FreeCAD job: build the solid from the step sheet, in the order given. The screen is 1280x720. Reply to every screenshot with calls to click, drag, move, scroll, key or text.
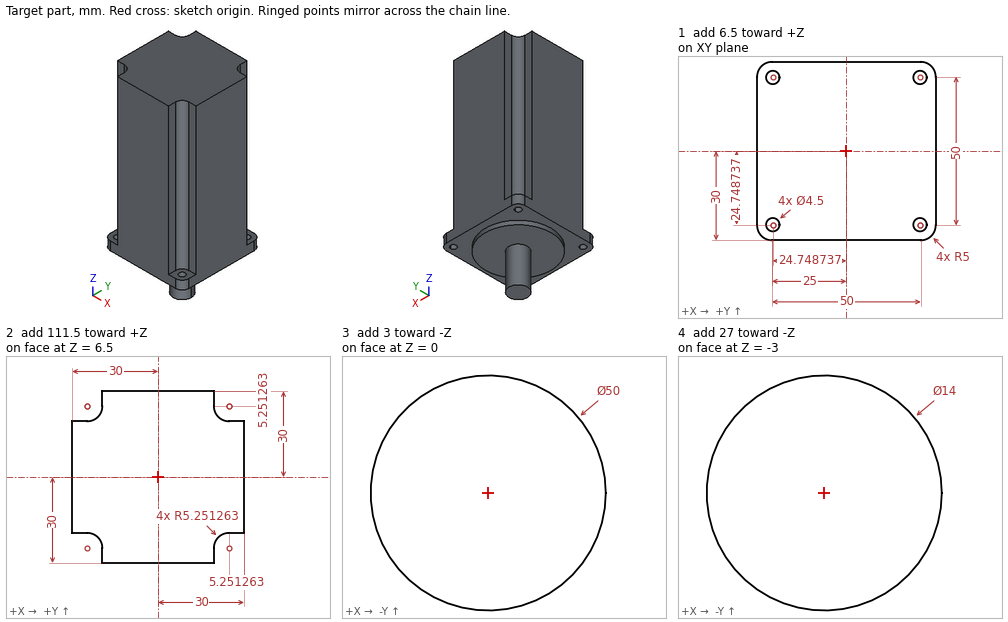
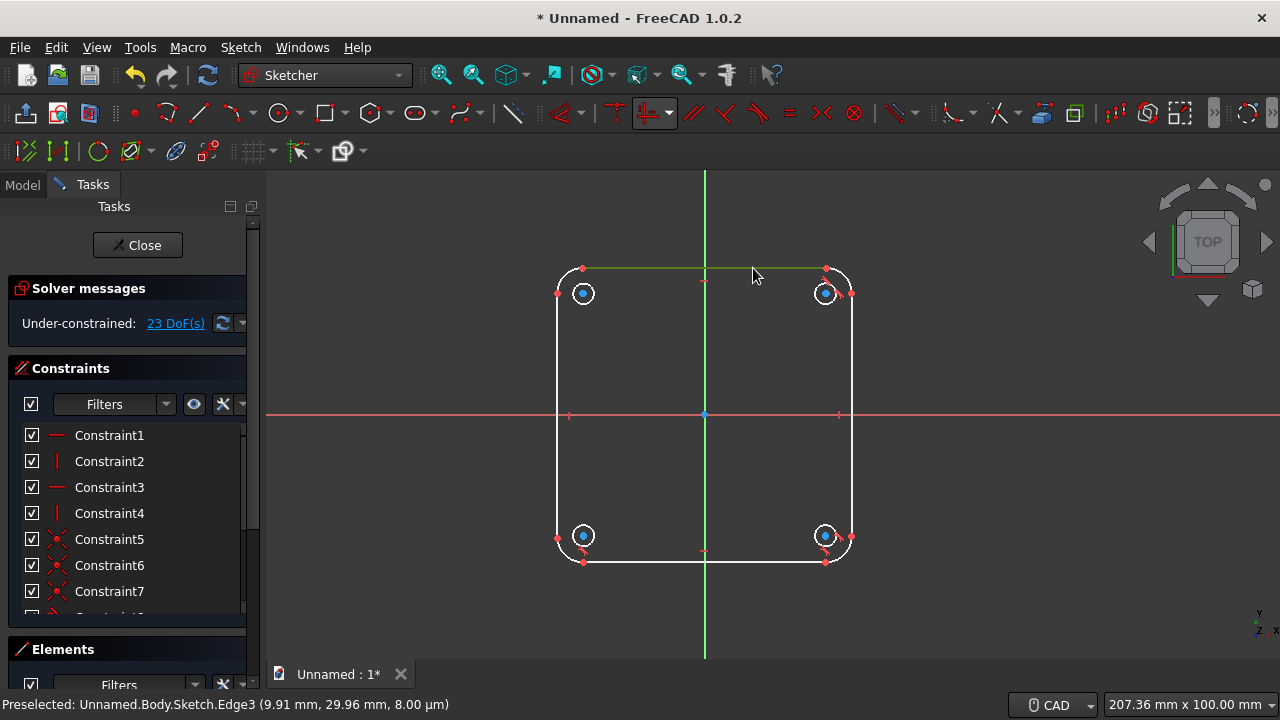
click(571, 271)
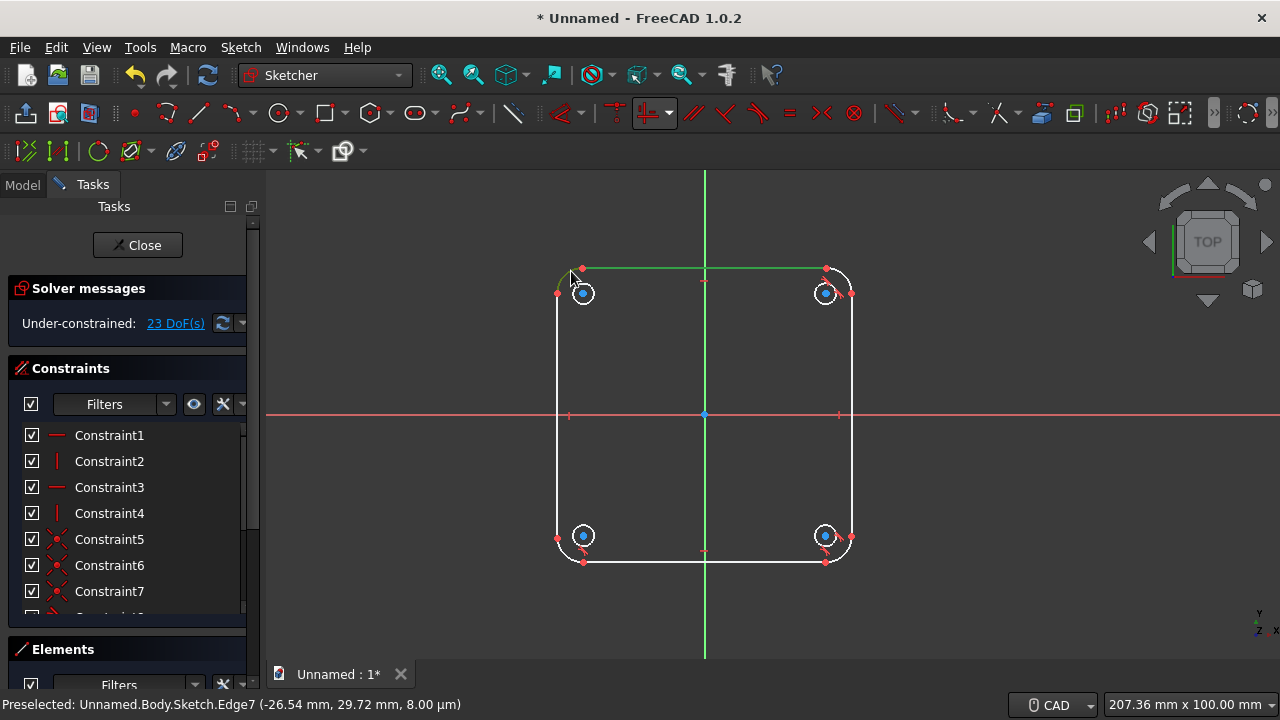
key(t)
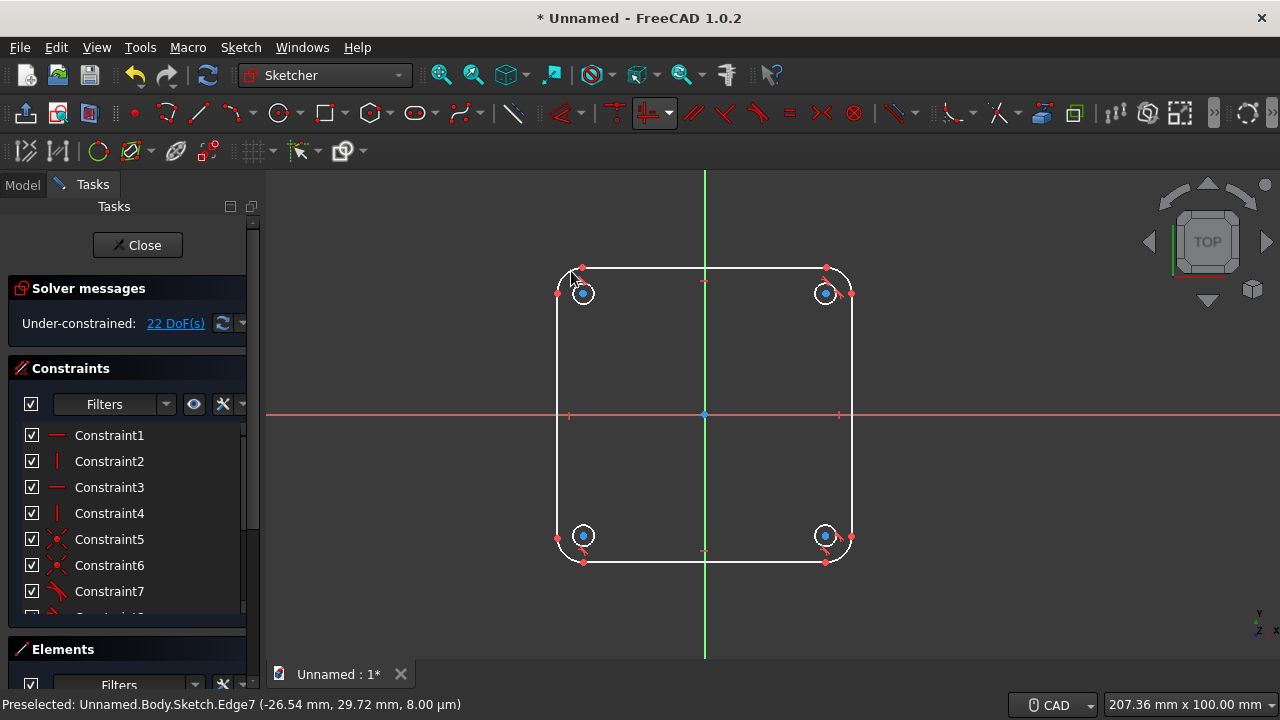
click(557, 367)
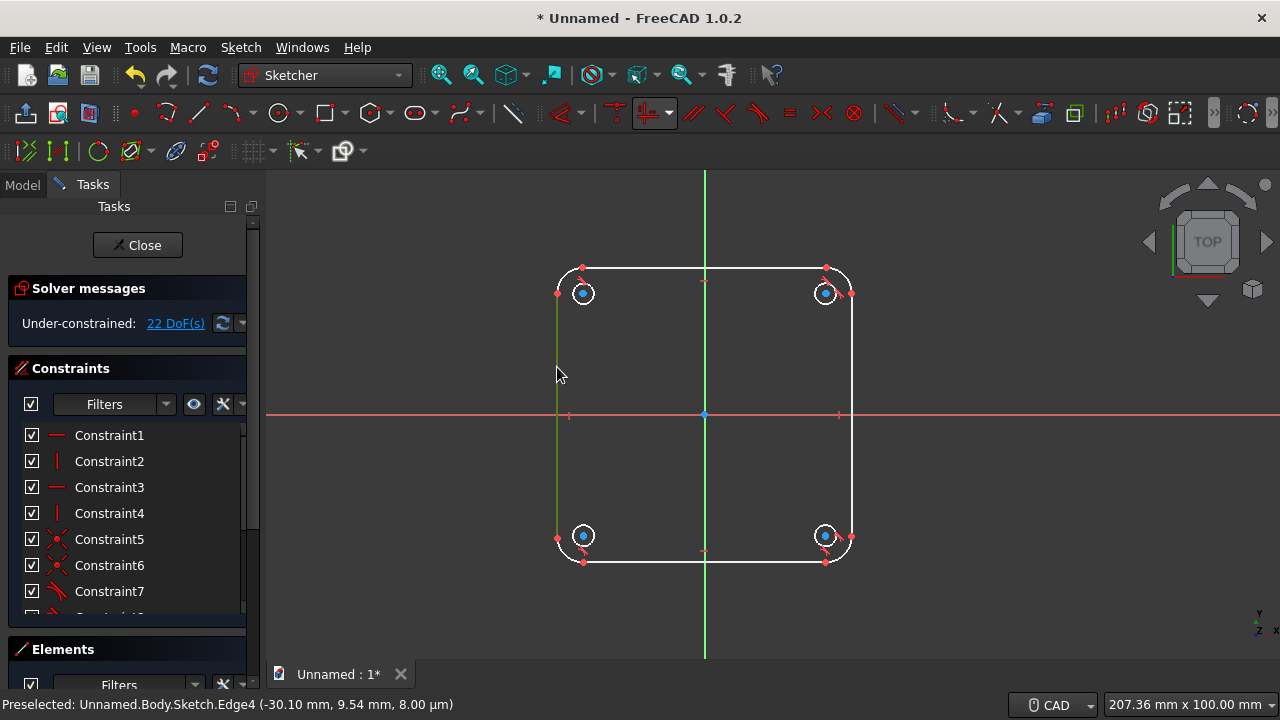
click(571, 271)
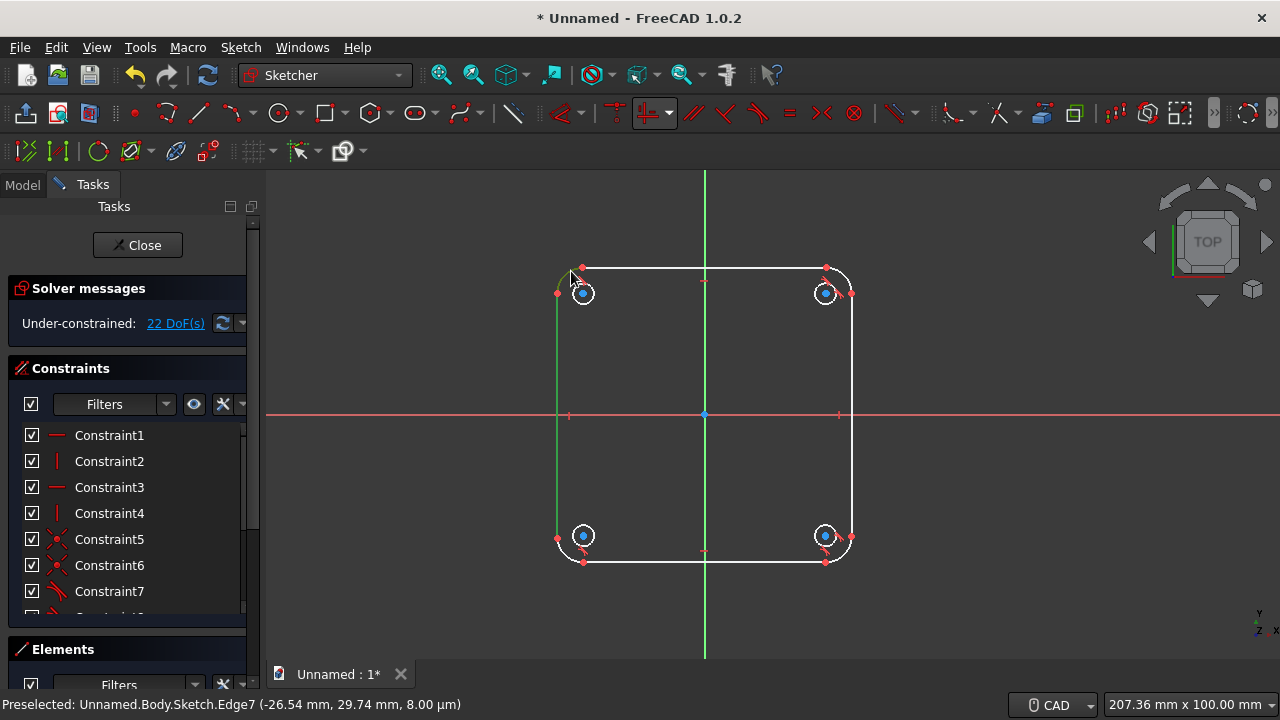
key(t)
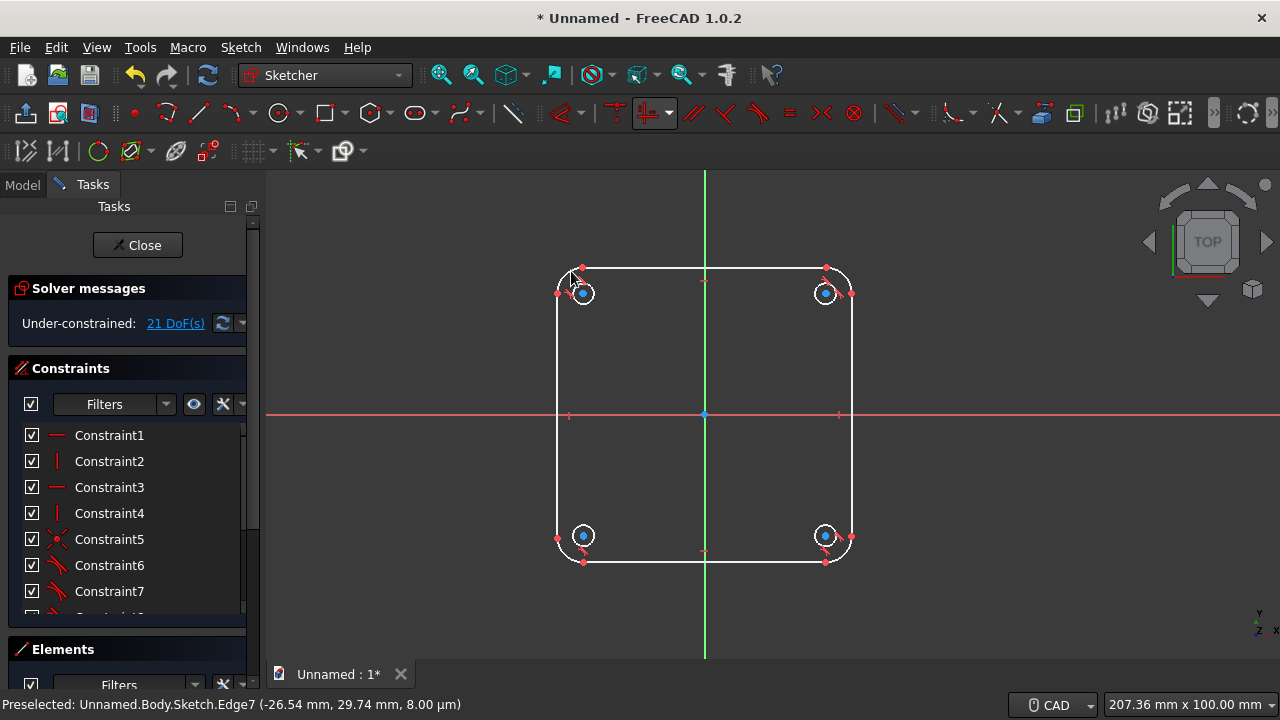
click(557, 367)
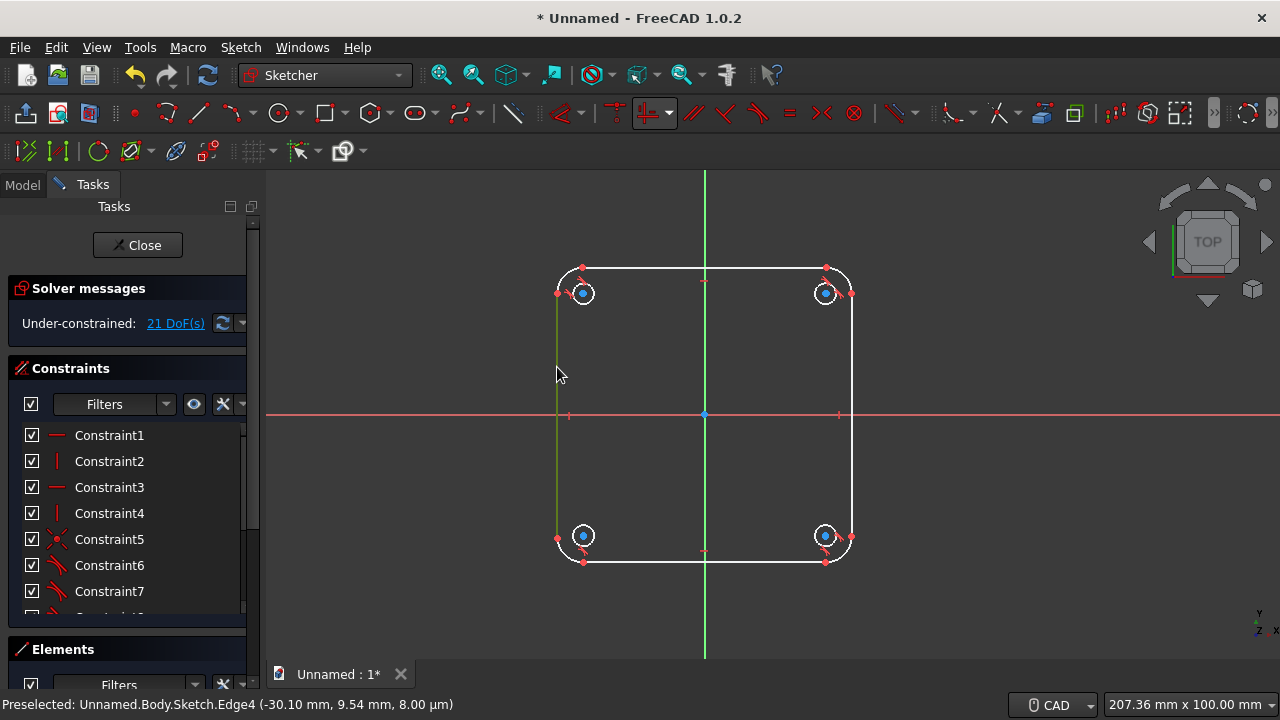
click(561, 549)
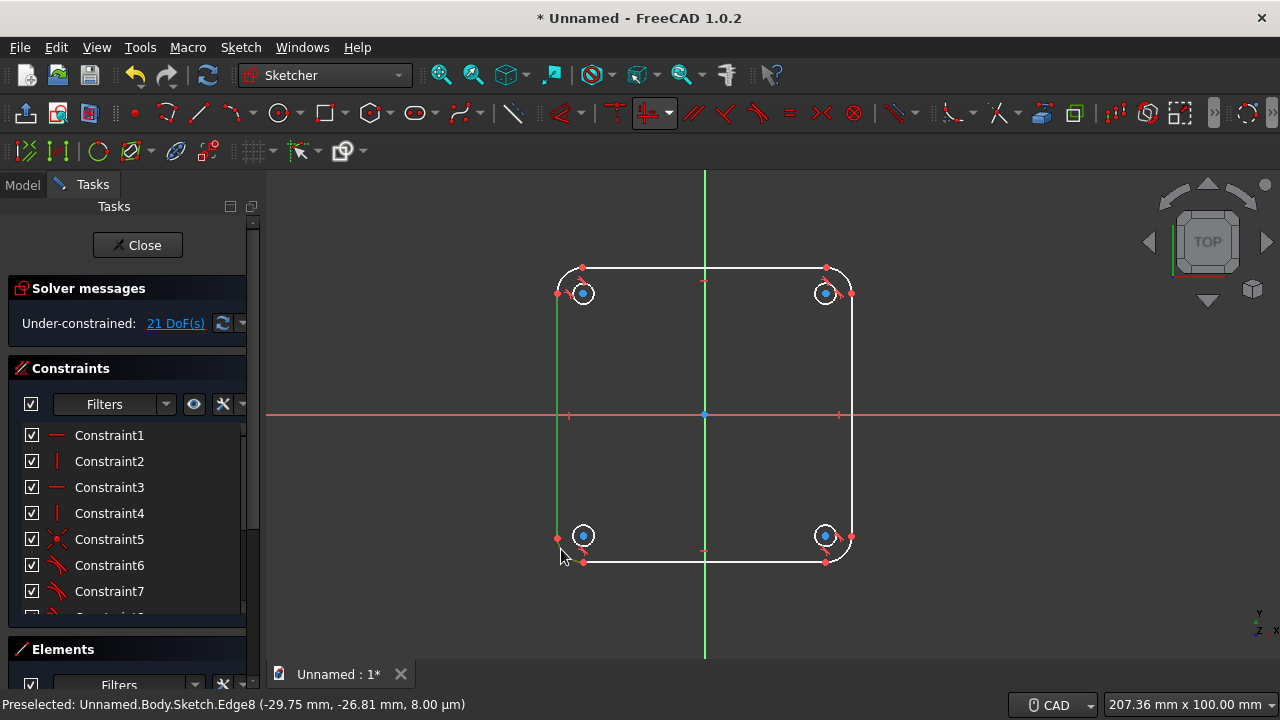
click(758, 114)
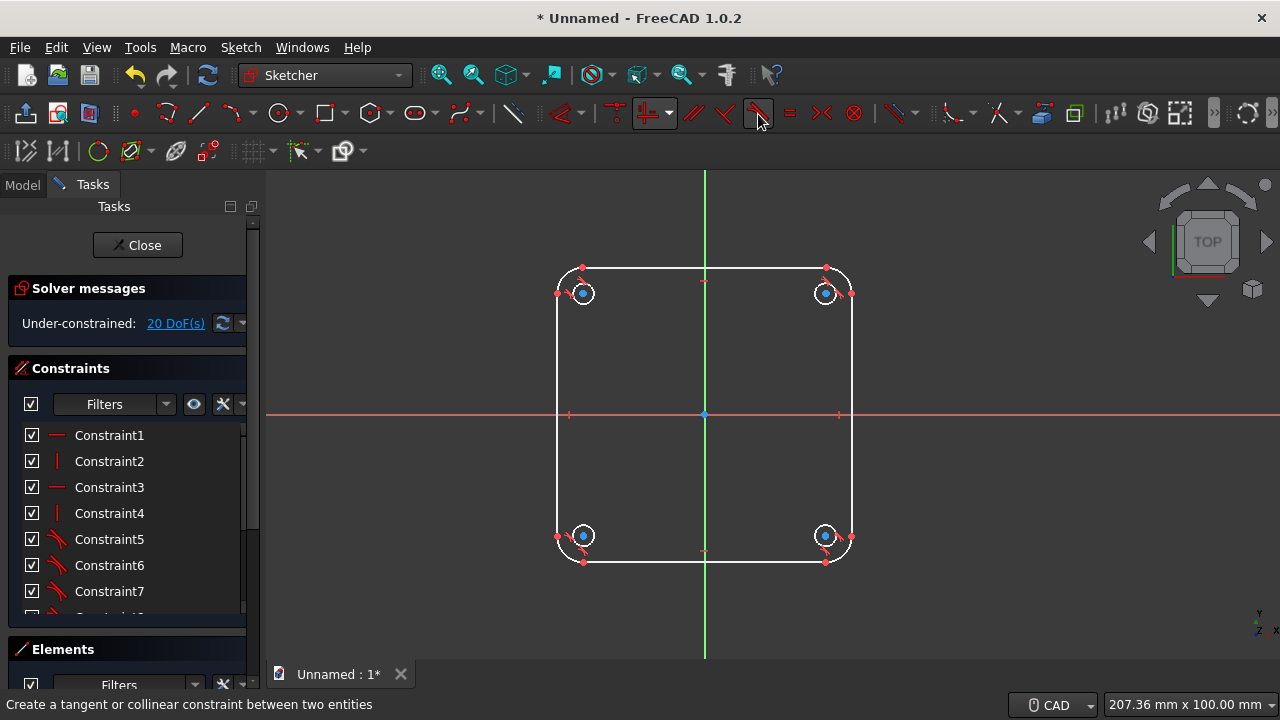
click(837, 559)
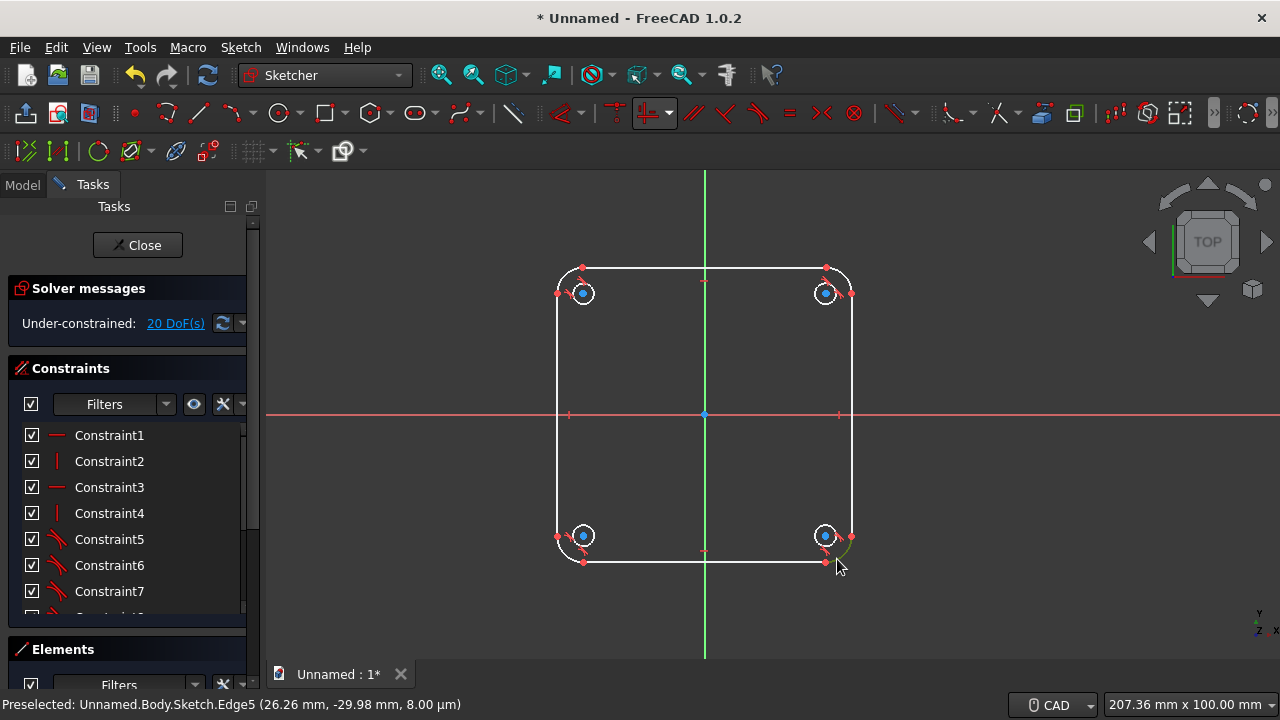
click(849, 282)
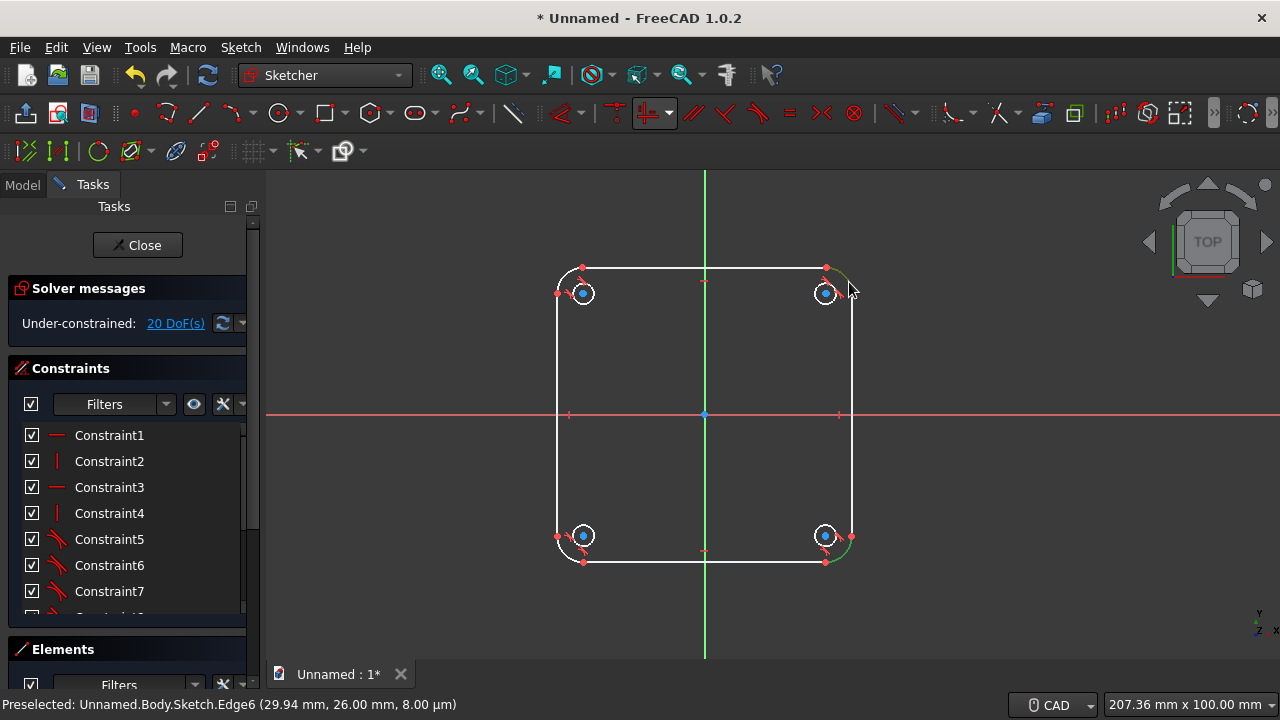
click(571, 271)